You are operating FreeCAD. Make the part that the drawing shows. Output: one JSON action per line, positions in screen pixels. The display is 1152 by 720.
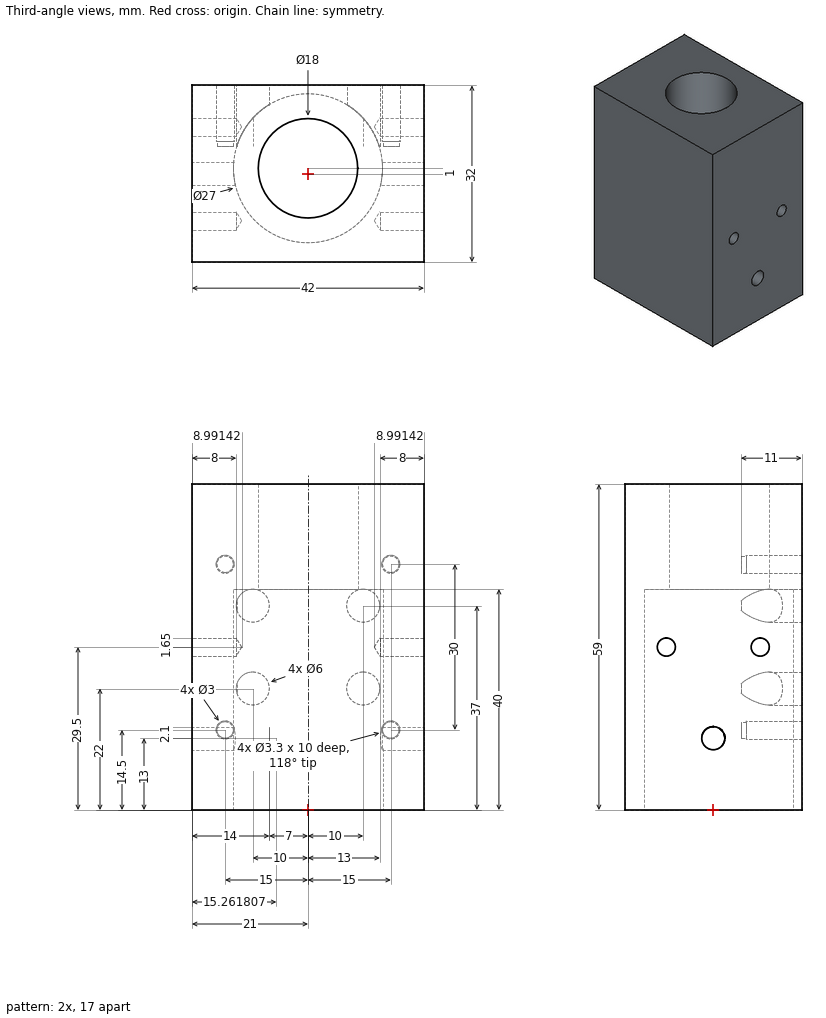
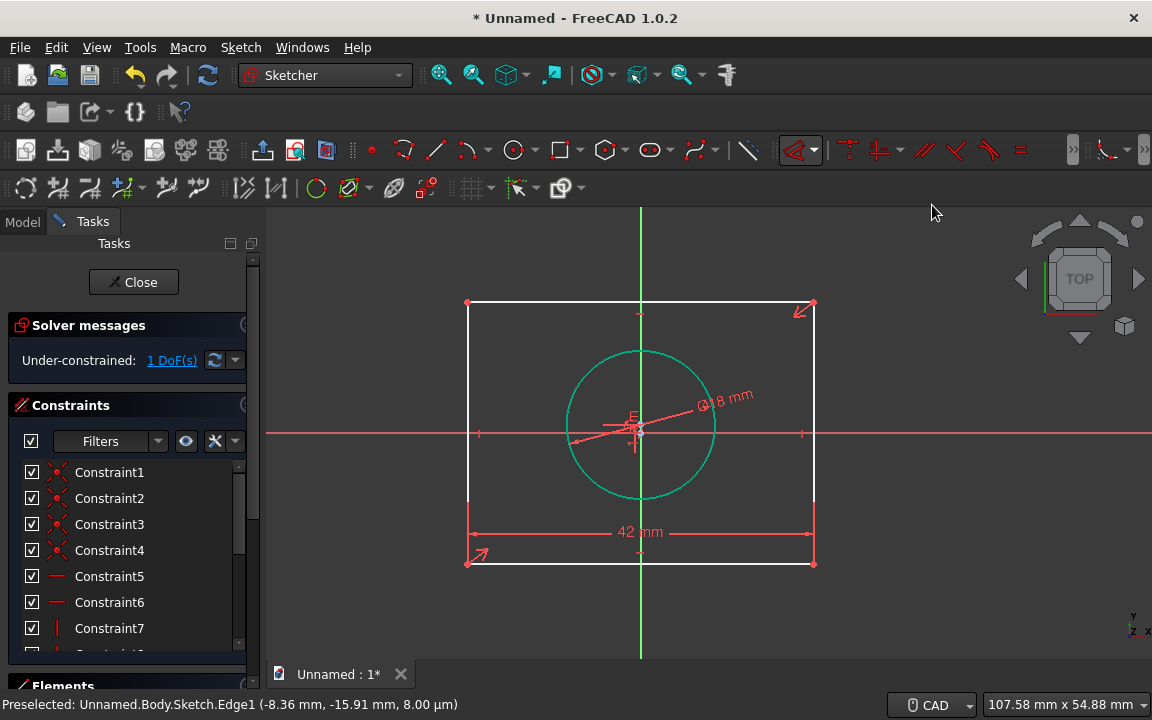
{"action": "left_click", "coordinate": [814, 486]}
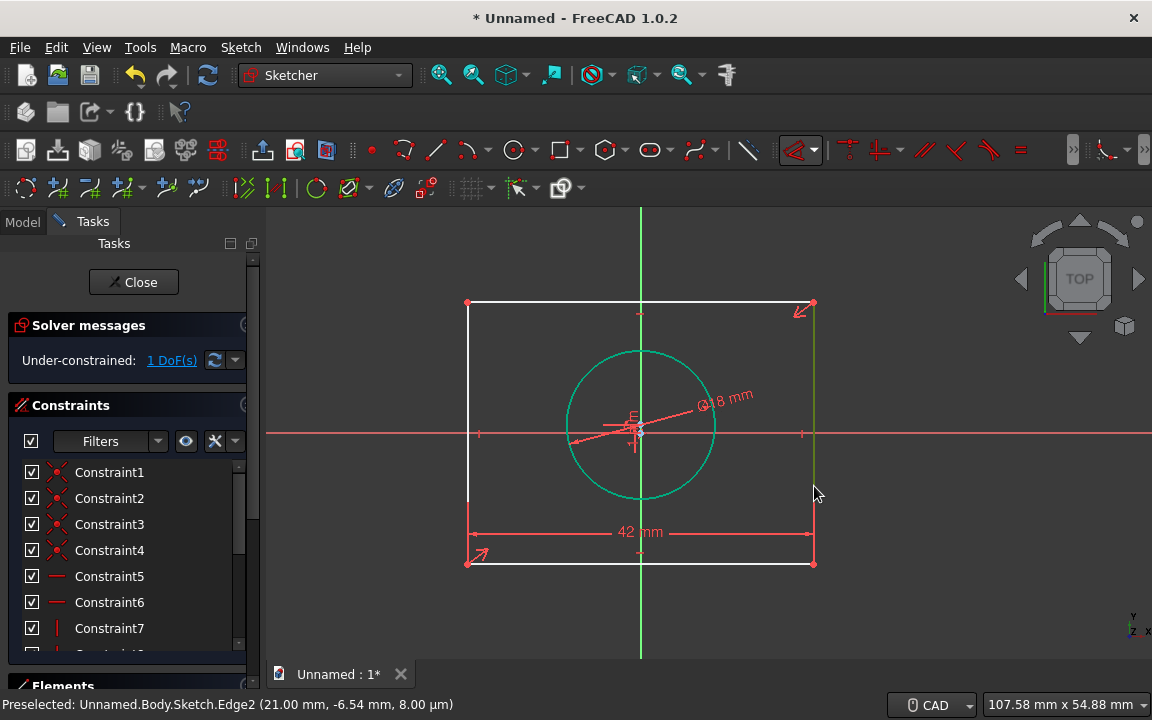
{"action": "left_click", "coordinate": [816, 150]}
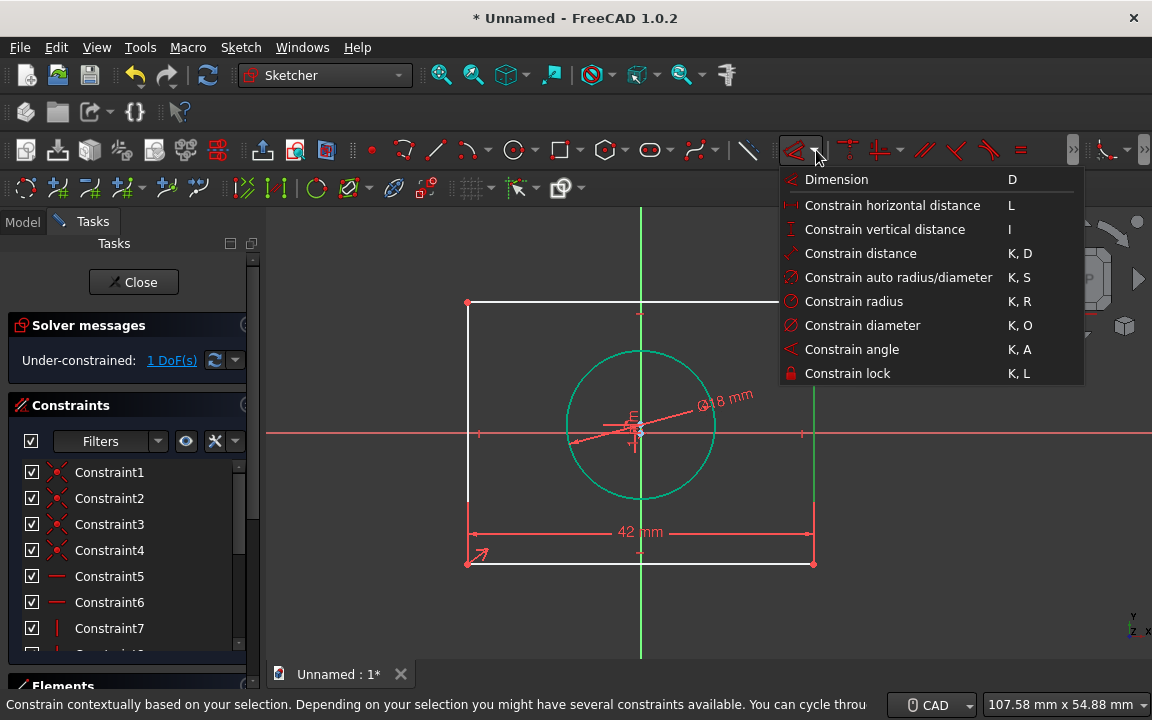
{"action": "left_click", "coordinate": [932, 229]}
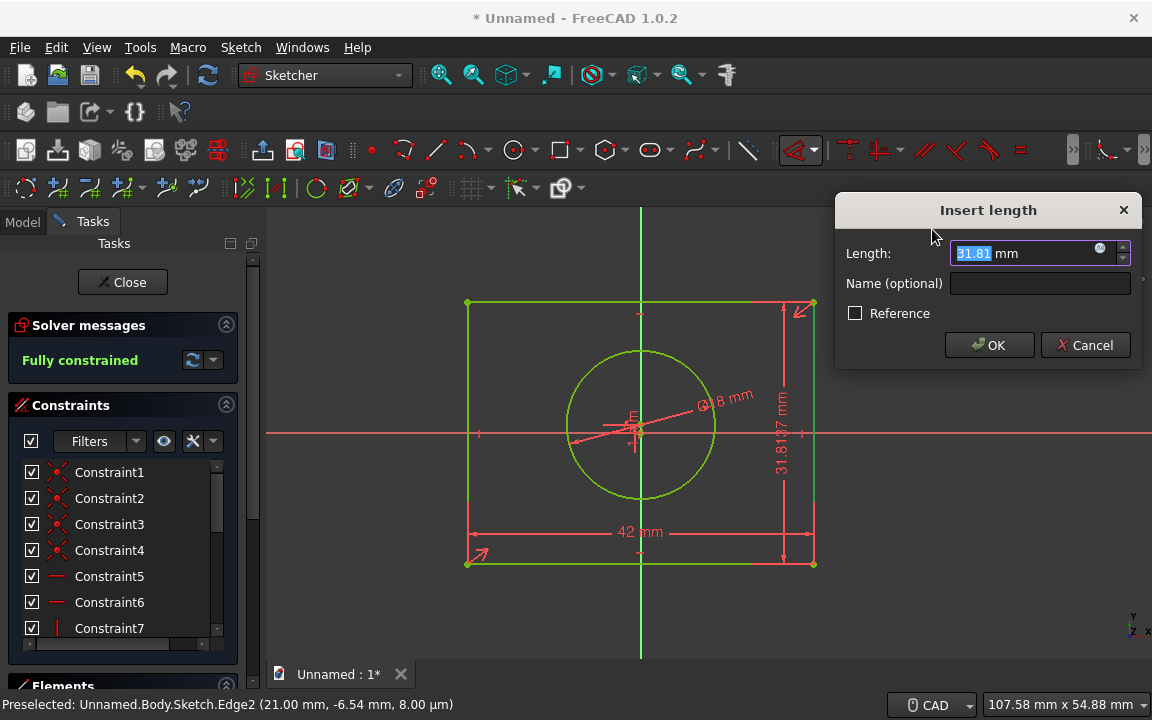
{"action": "type", "text": "32"}
{"action": "key", "text": "Return"}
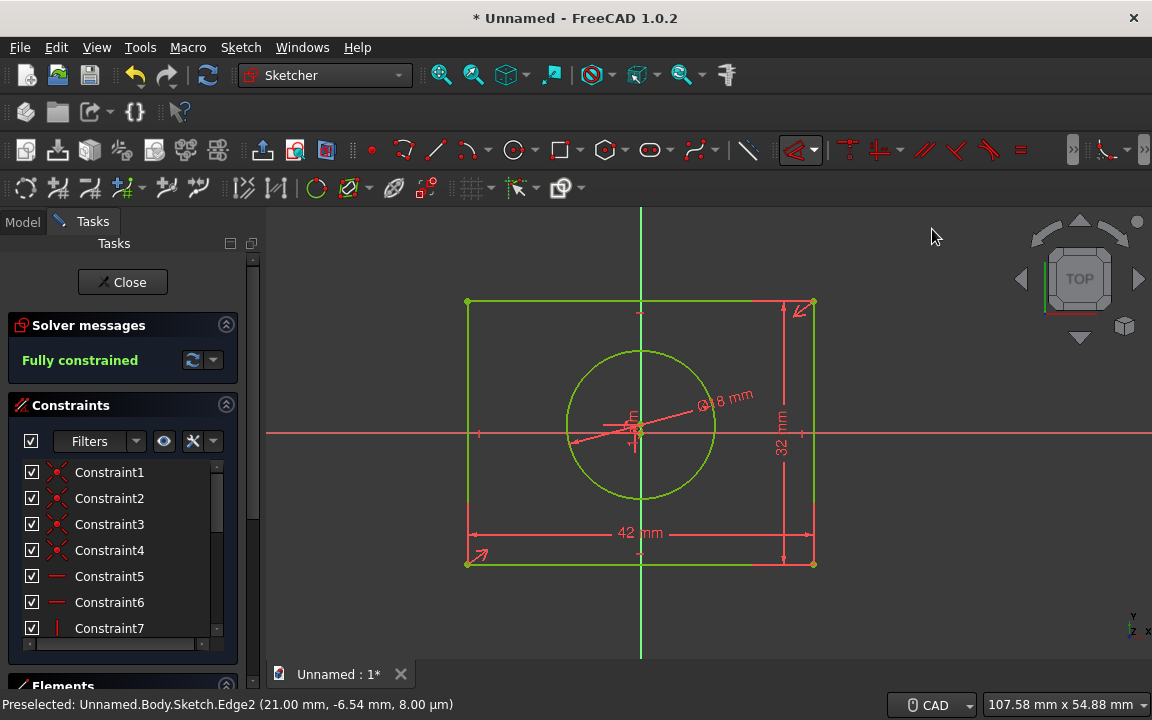
{"action": "left_click", "coordinate": [123, 282]}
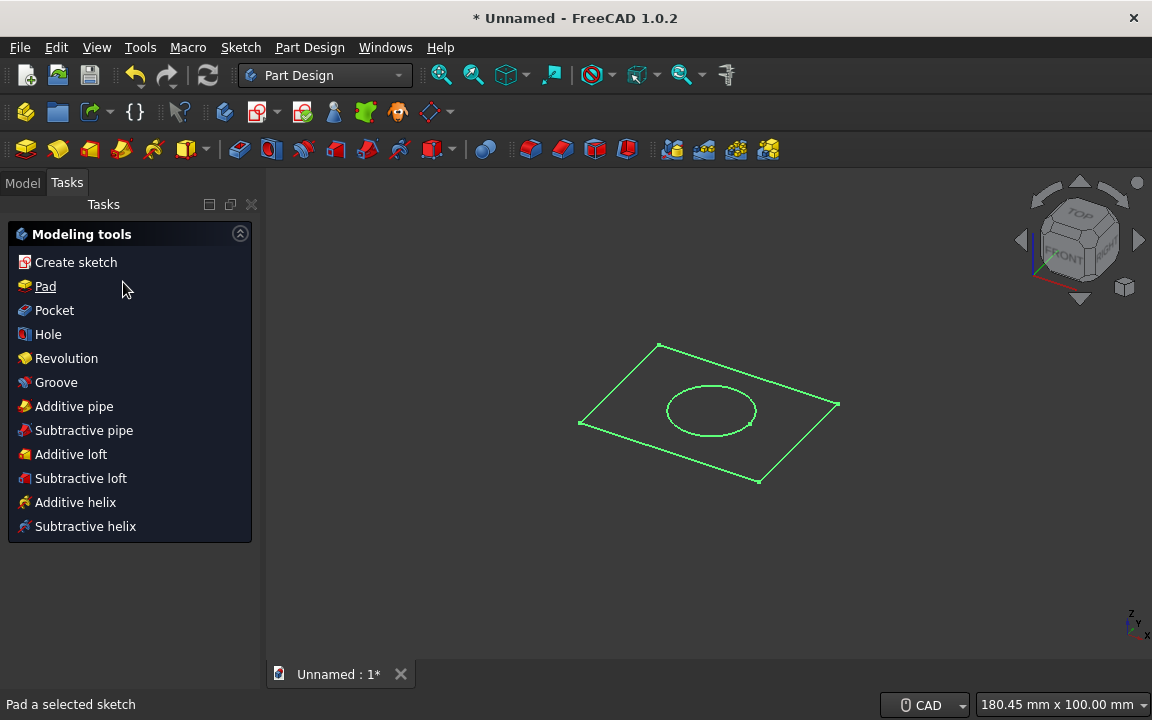
{"action": "left_click", "coordinate": [26, 150]}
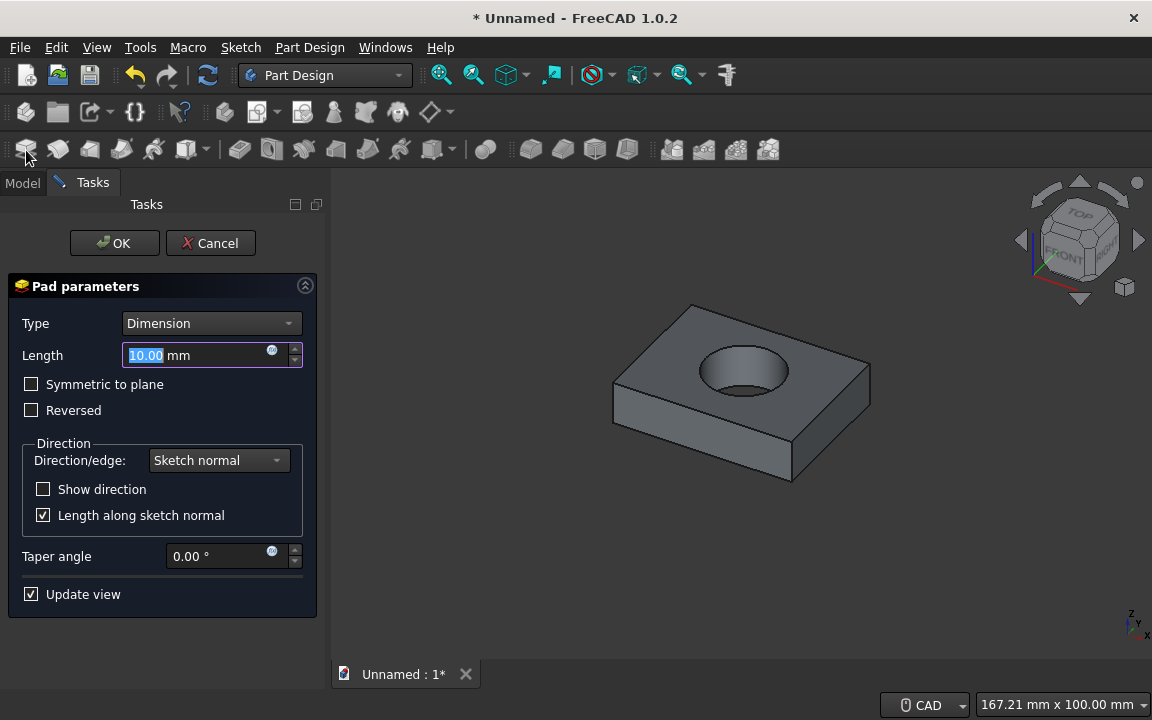
{"action": "type", "text": "59"}
{"action": "key", "text": "Tab"}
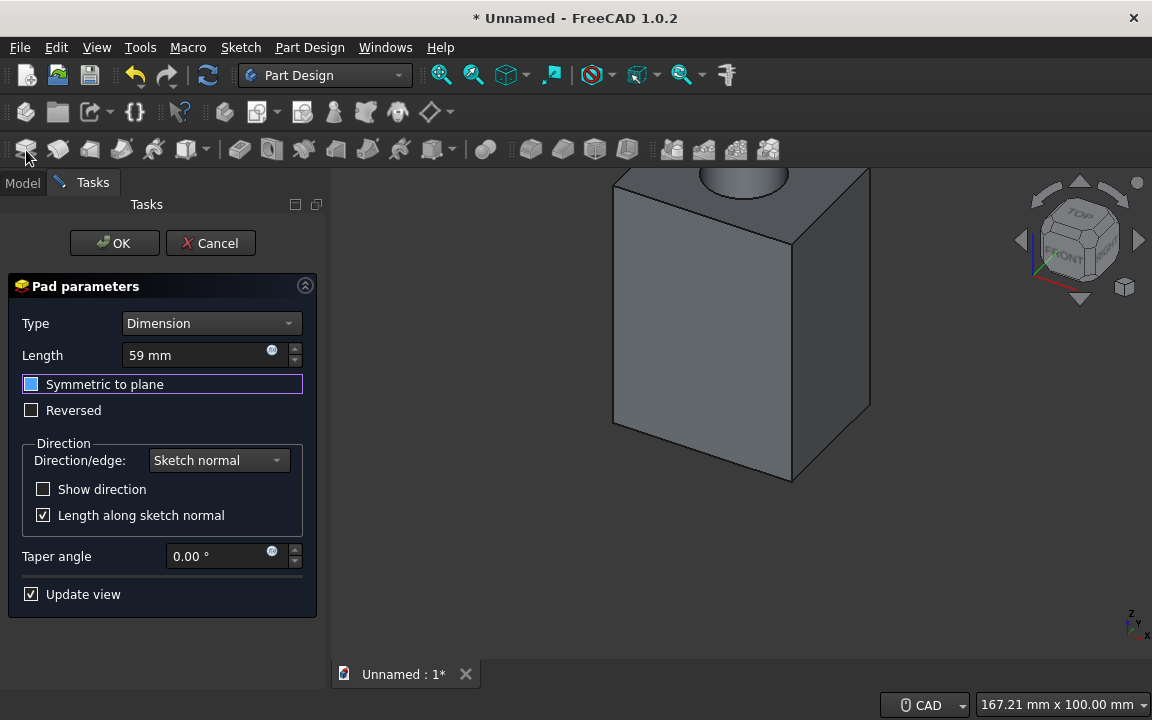
{"action": "left_click", "coordinate": [115, 243]}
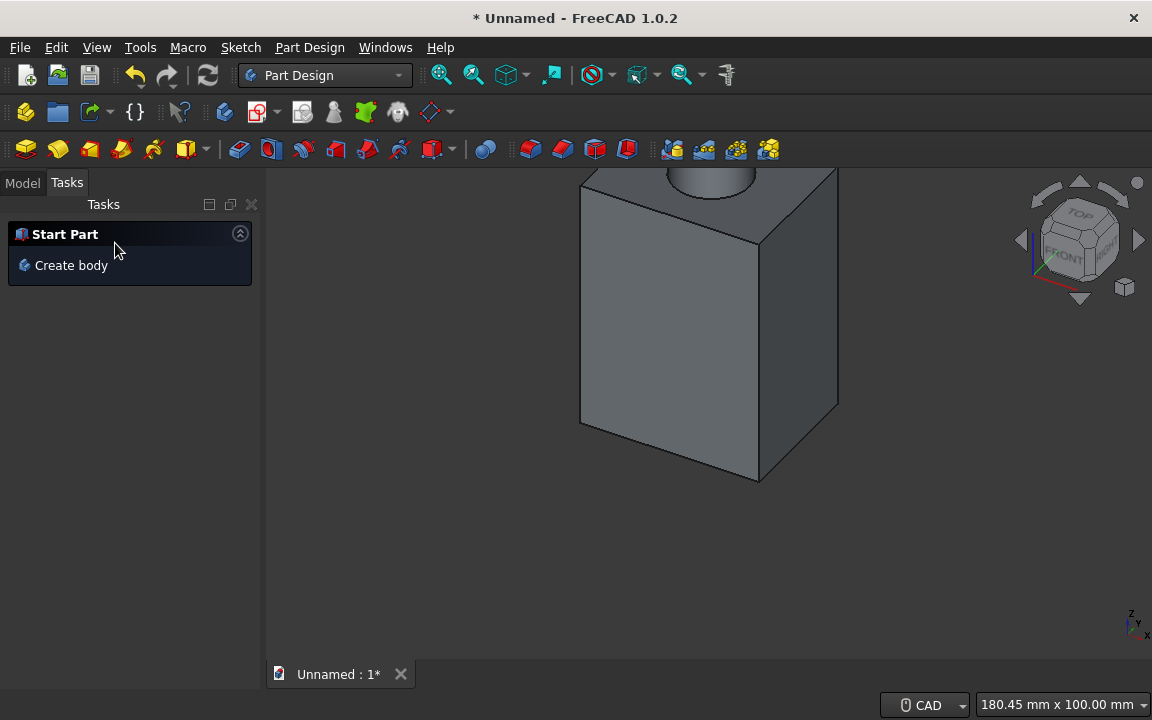
{"action": "left_click", "coordinate": [442, 76]}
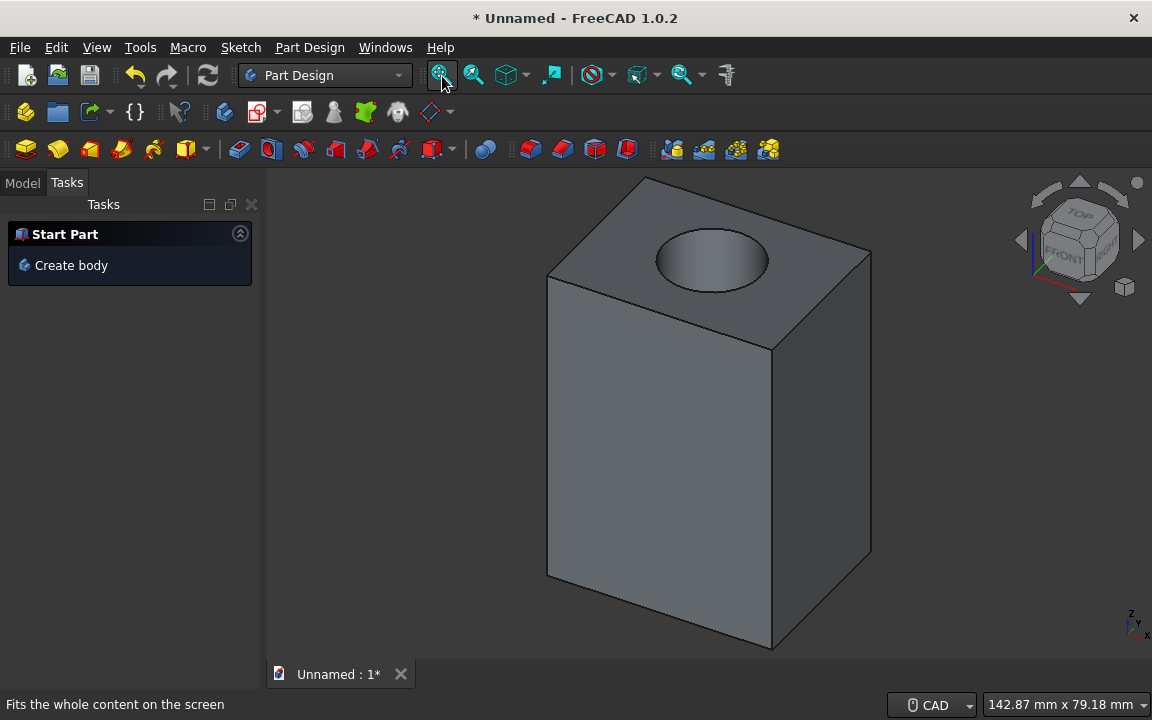
{"action": "left_click", "coordinate": [258, 112]}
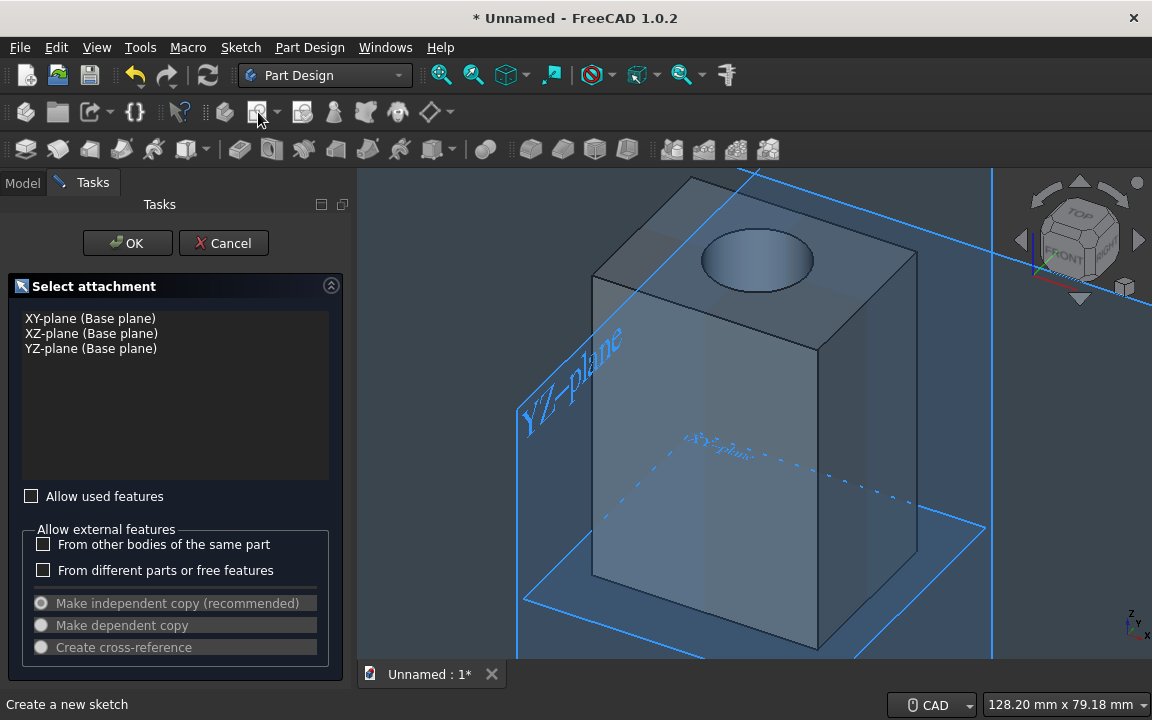
{"action": "left_click", "coordinate": [82, 318]}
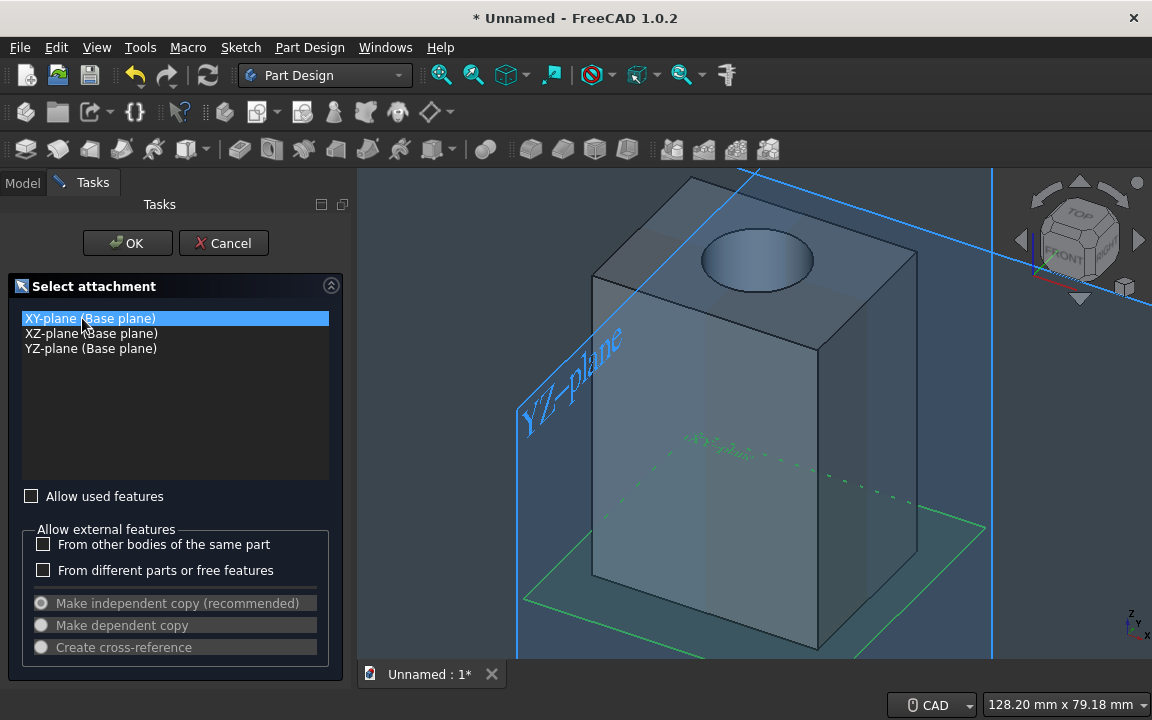
{"action": "left_click", "coordinate": [128, 243]}